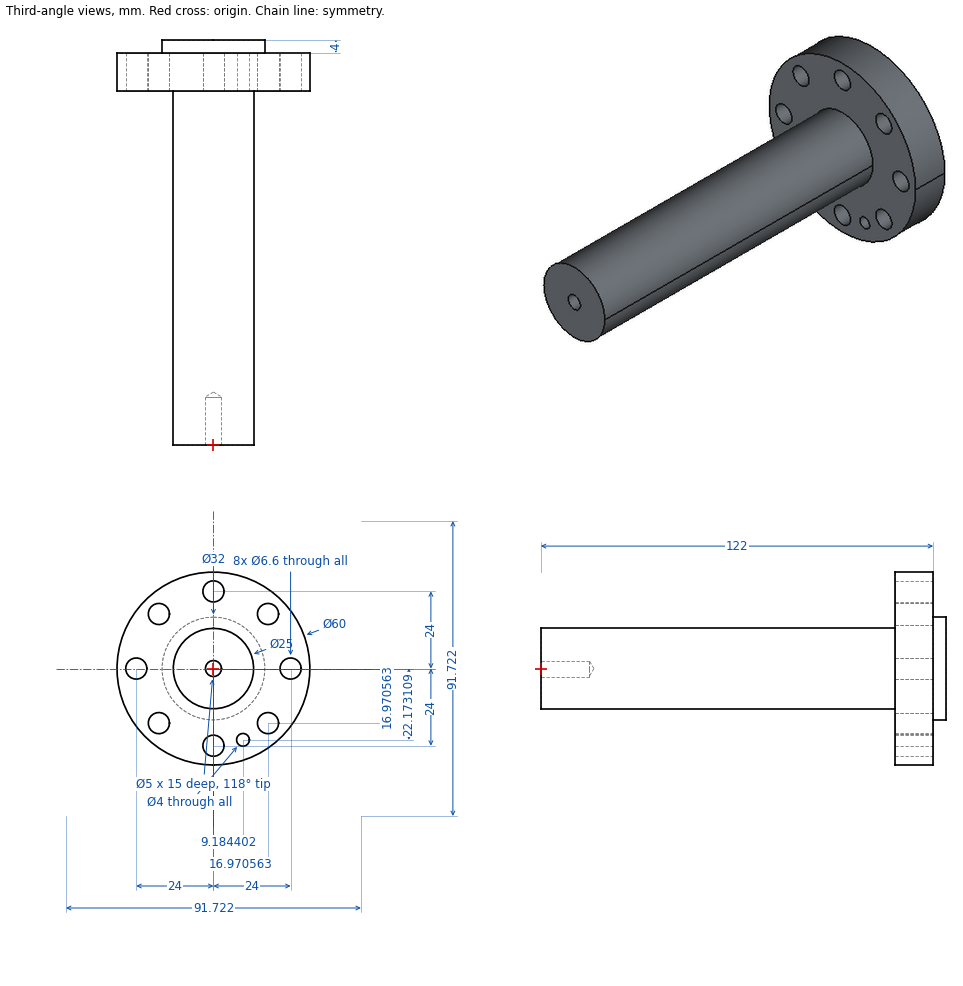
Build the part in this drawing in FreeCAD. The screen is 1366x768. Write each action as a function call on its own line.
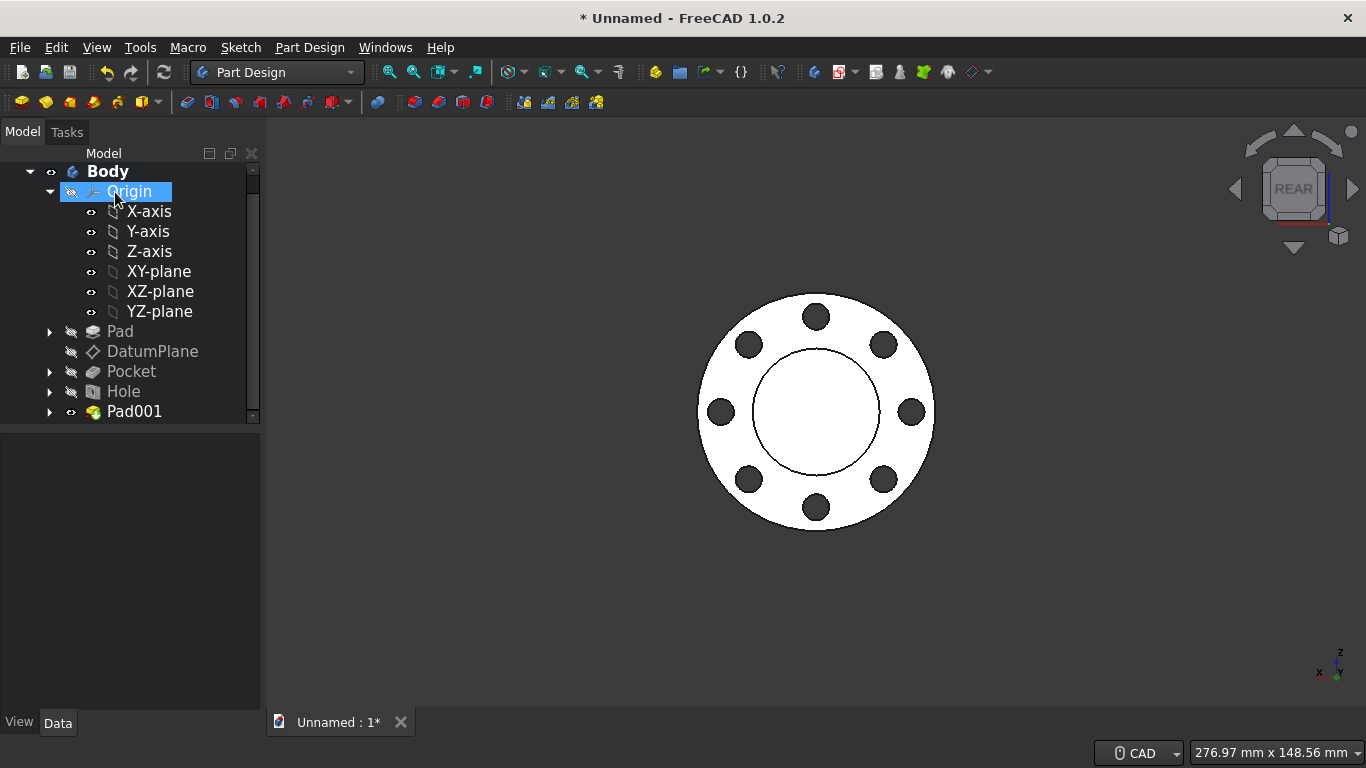
click(390, 72)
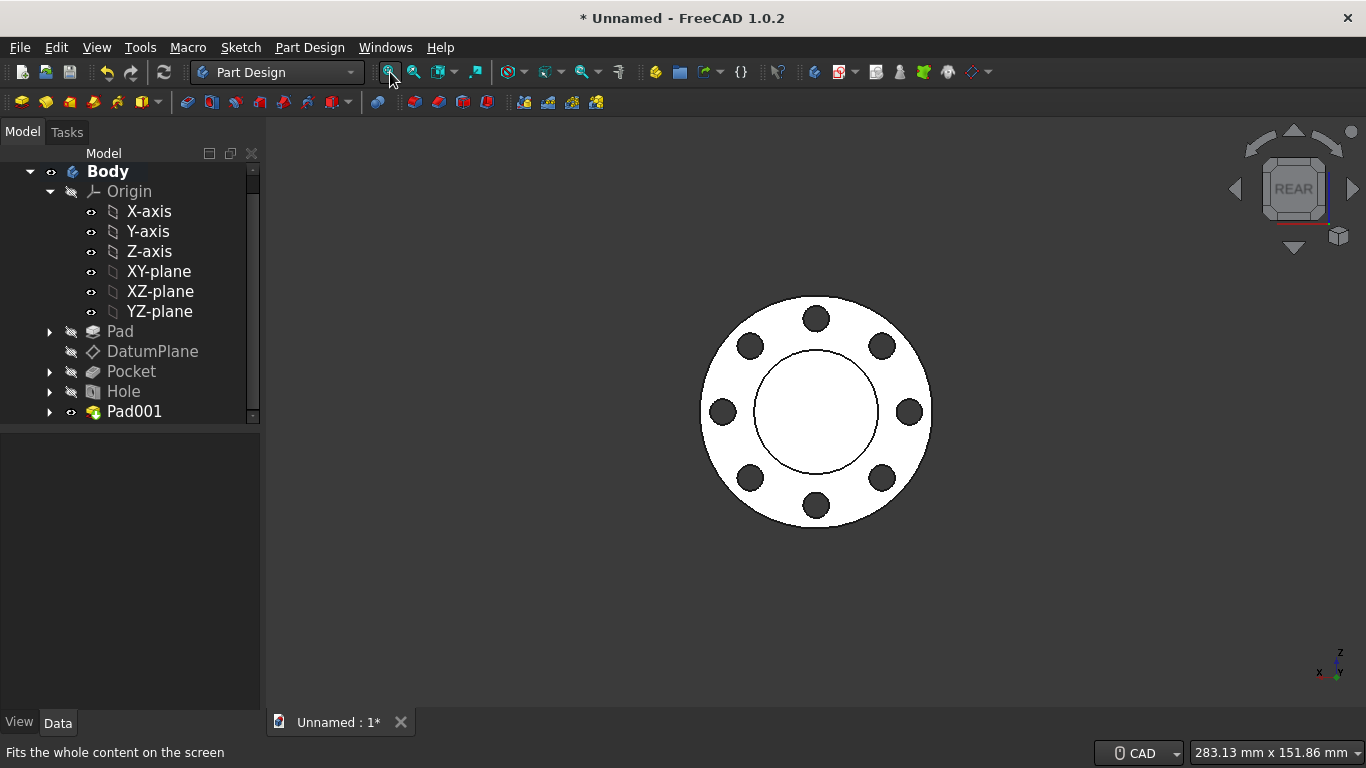
key(0)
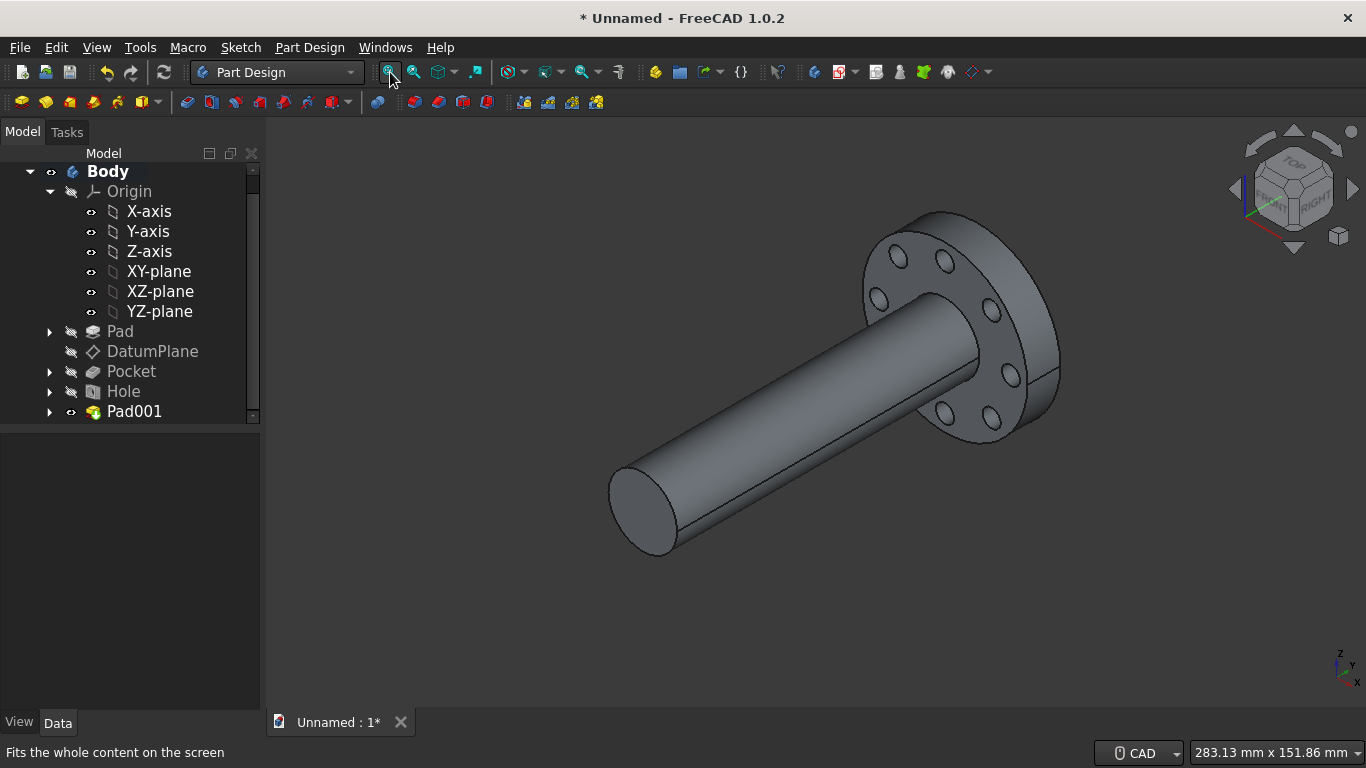
click(992, 391)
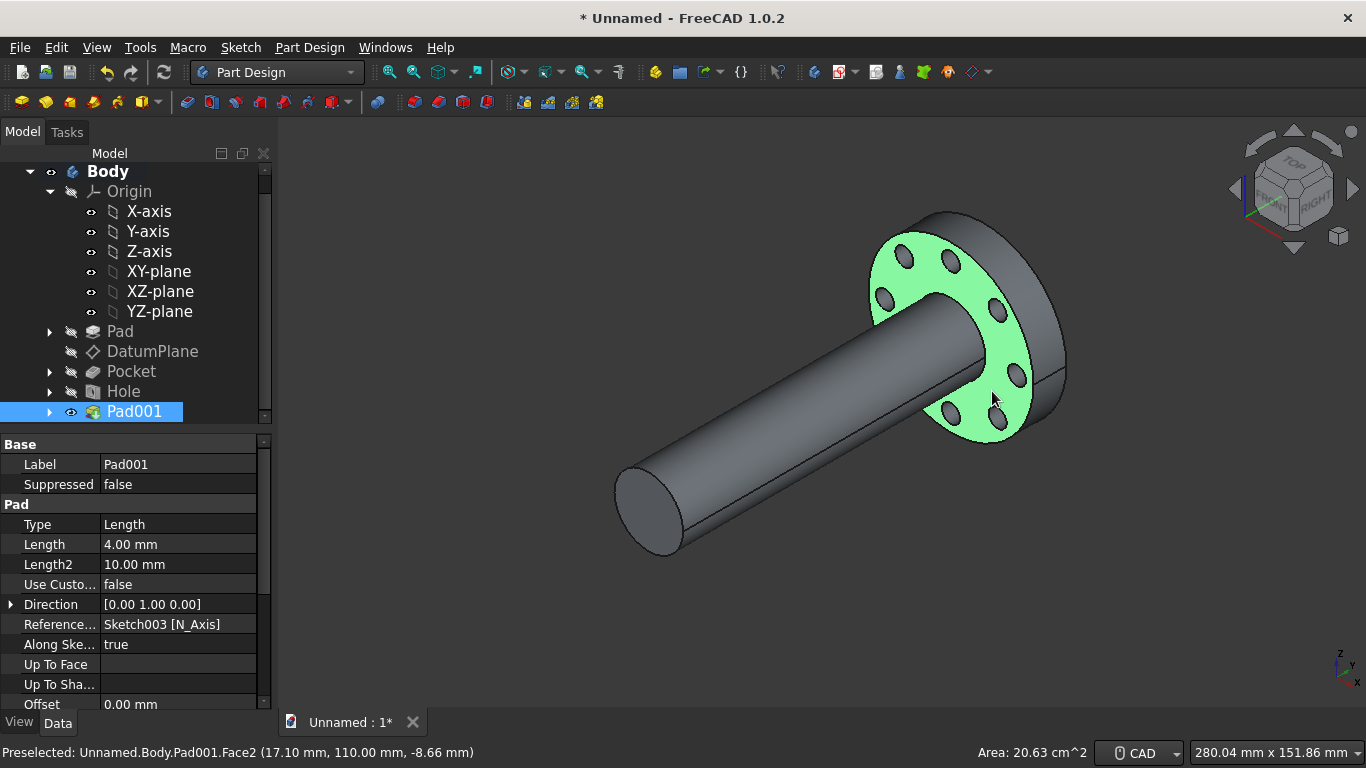
click(840, 72)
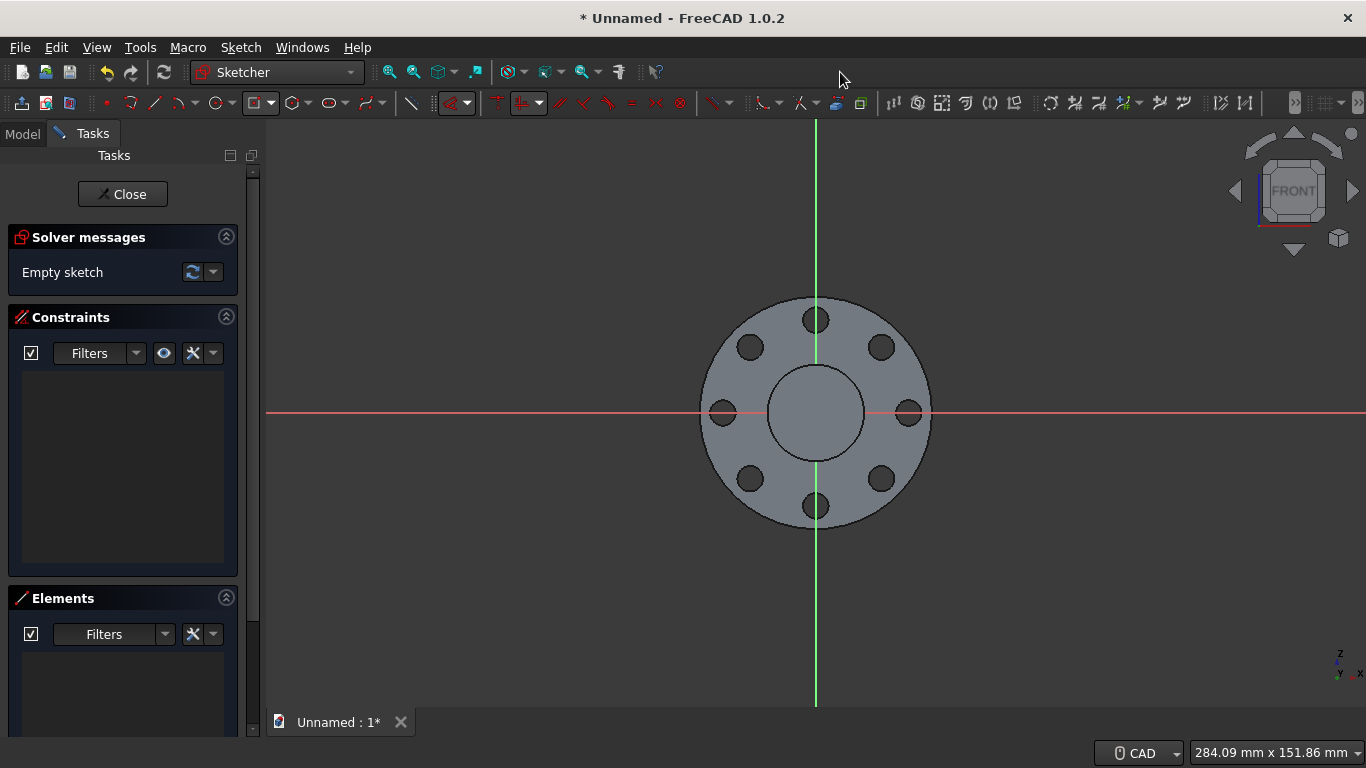
scroll(857, 503, up, 15)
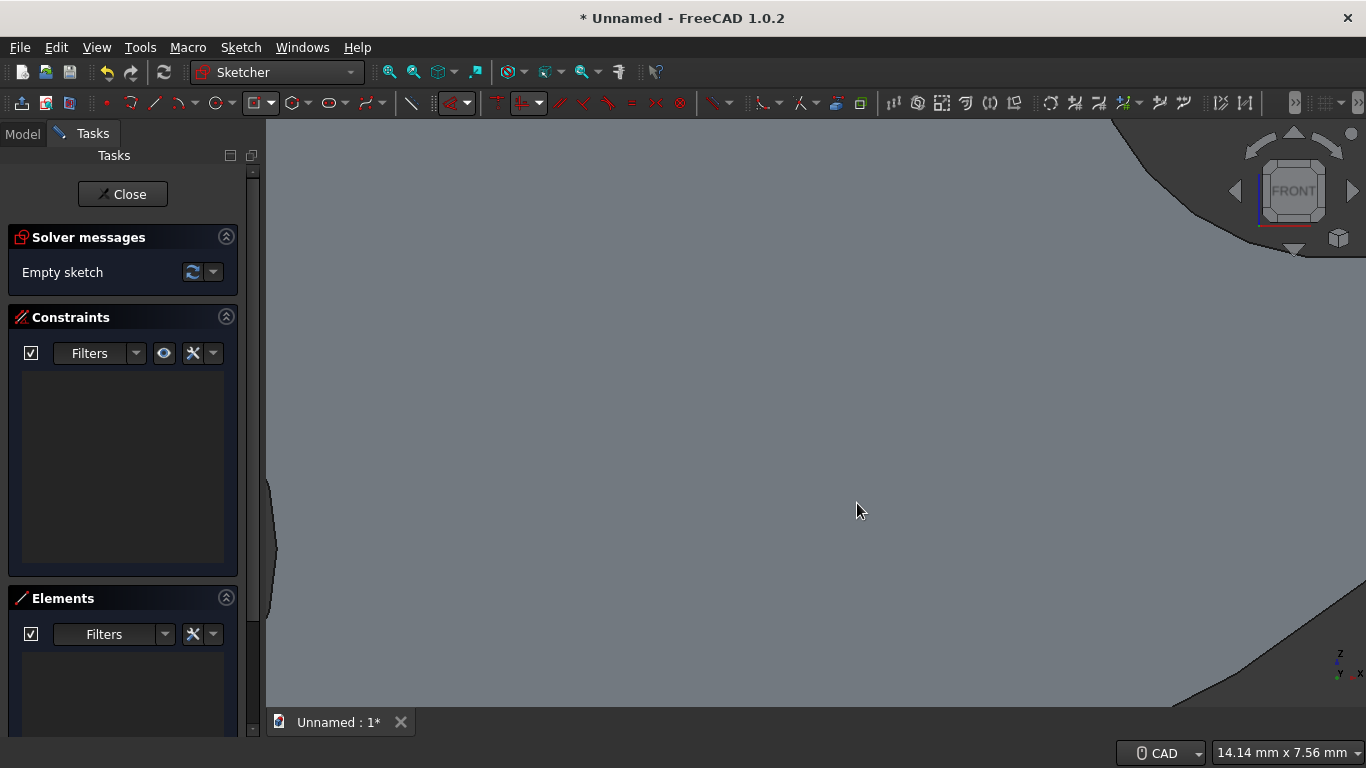
click(216, 104)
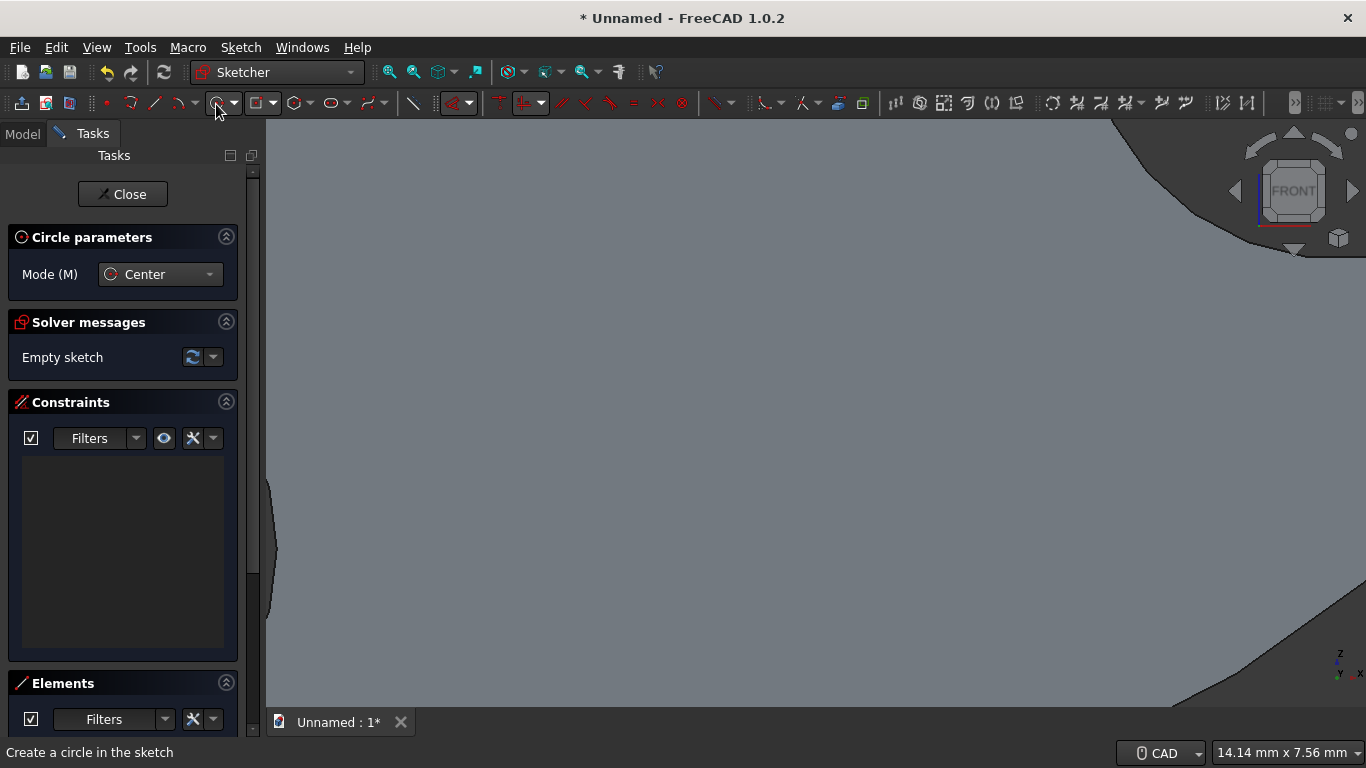
click(734, 407)
click(844, 297)
key(Escape)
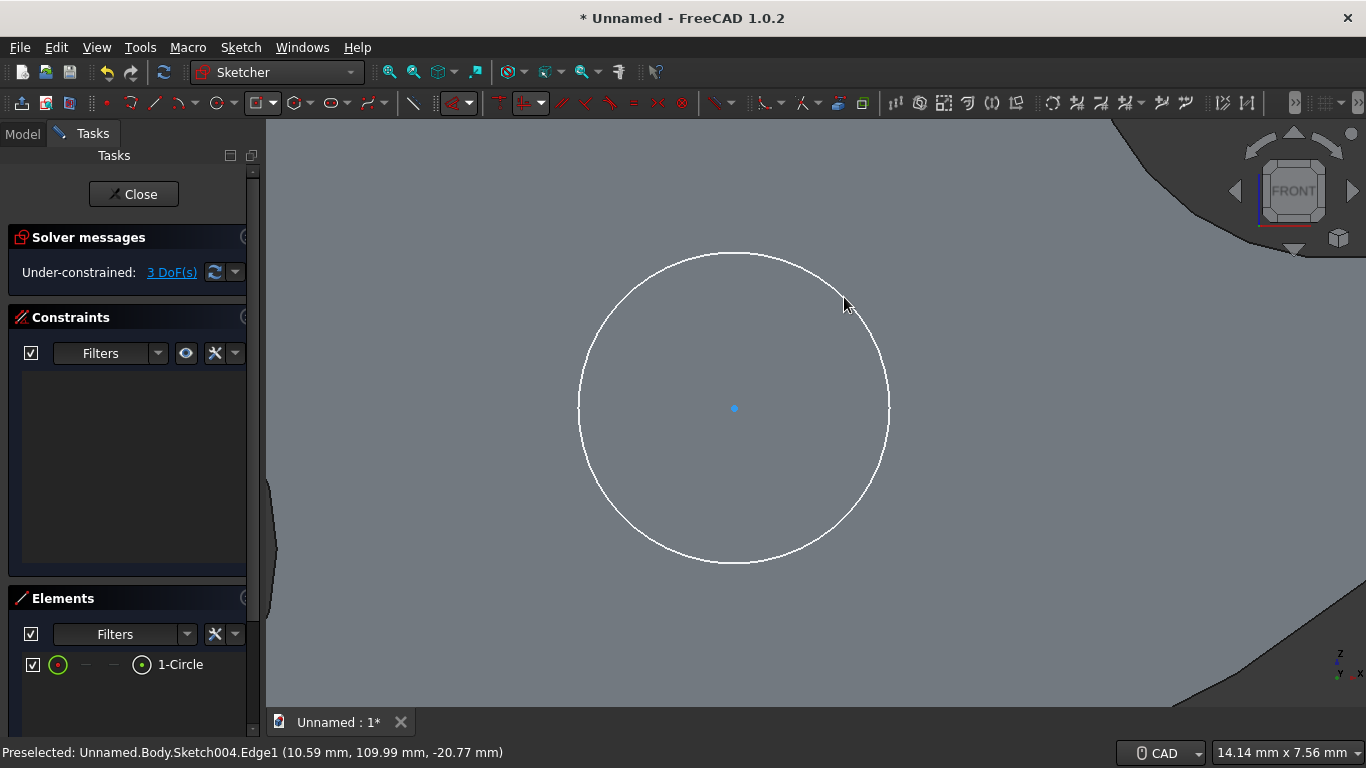
click(844, 298)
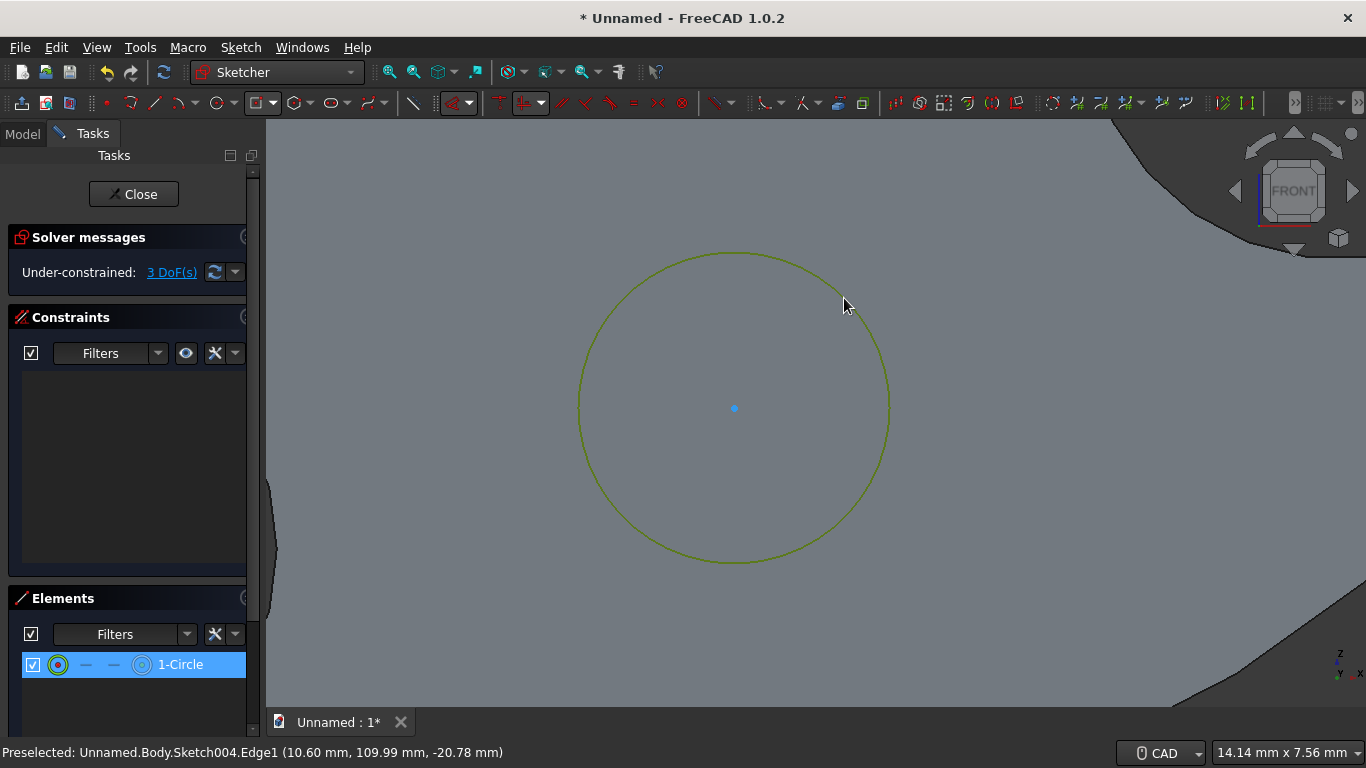
key(k)
key(o)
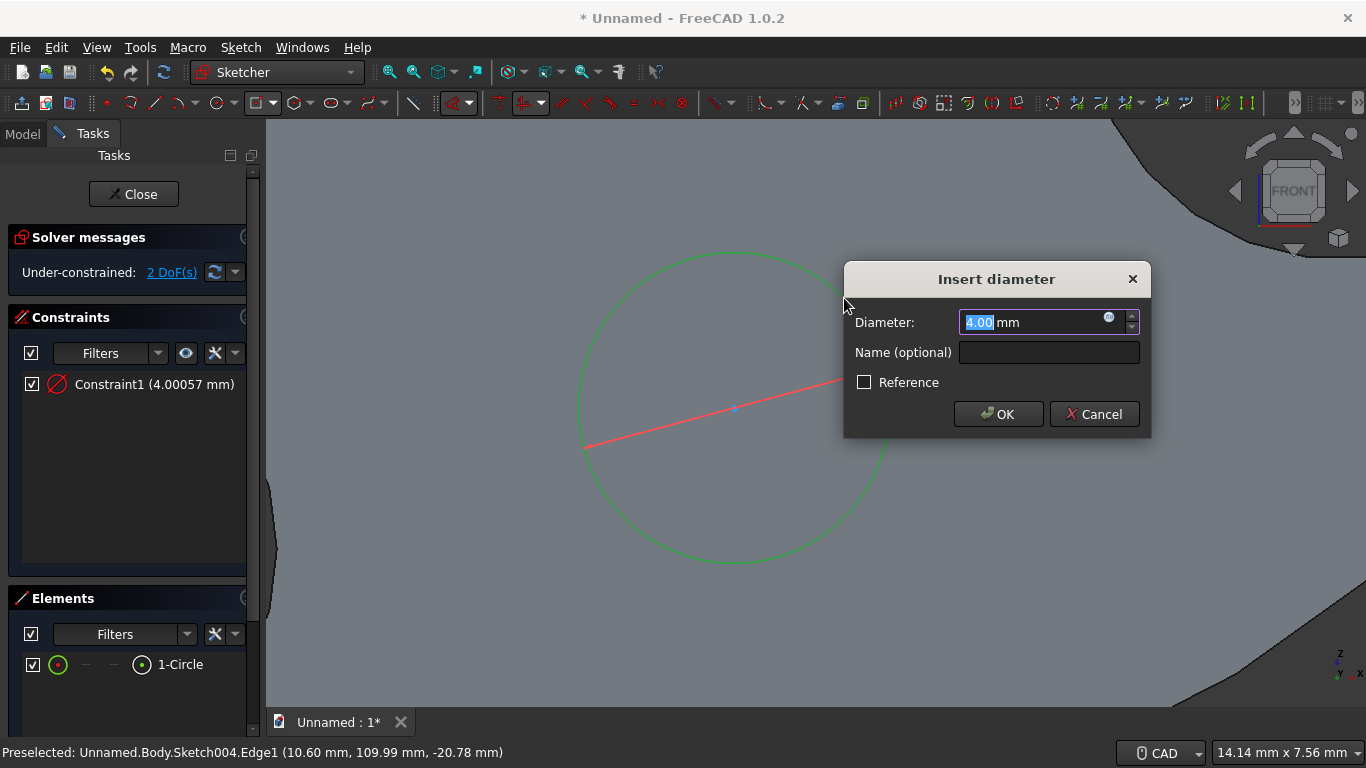
text(4)
key(Return)